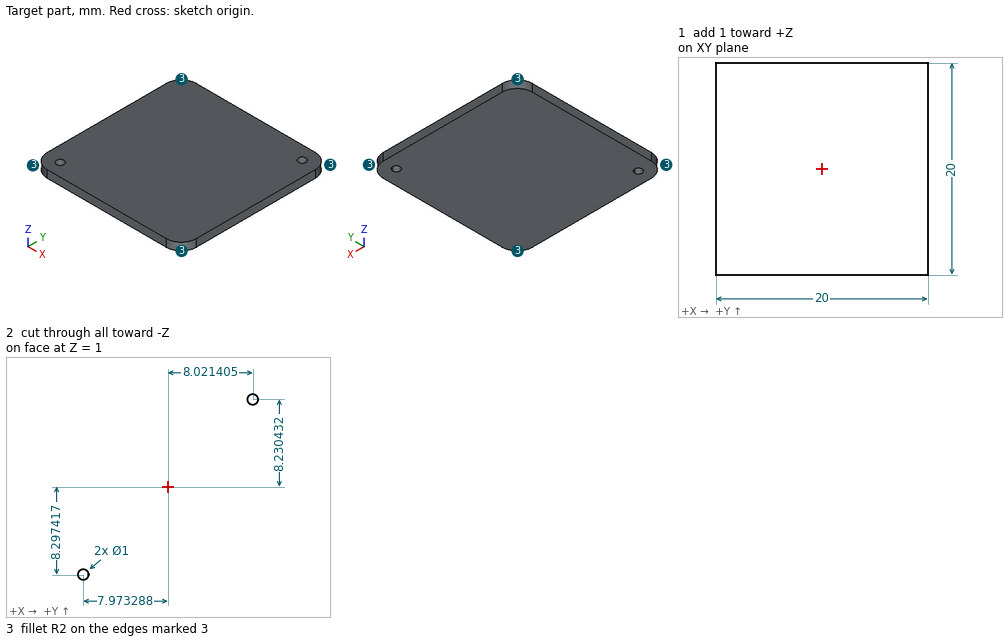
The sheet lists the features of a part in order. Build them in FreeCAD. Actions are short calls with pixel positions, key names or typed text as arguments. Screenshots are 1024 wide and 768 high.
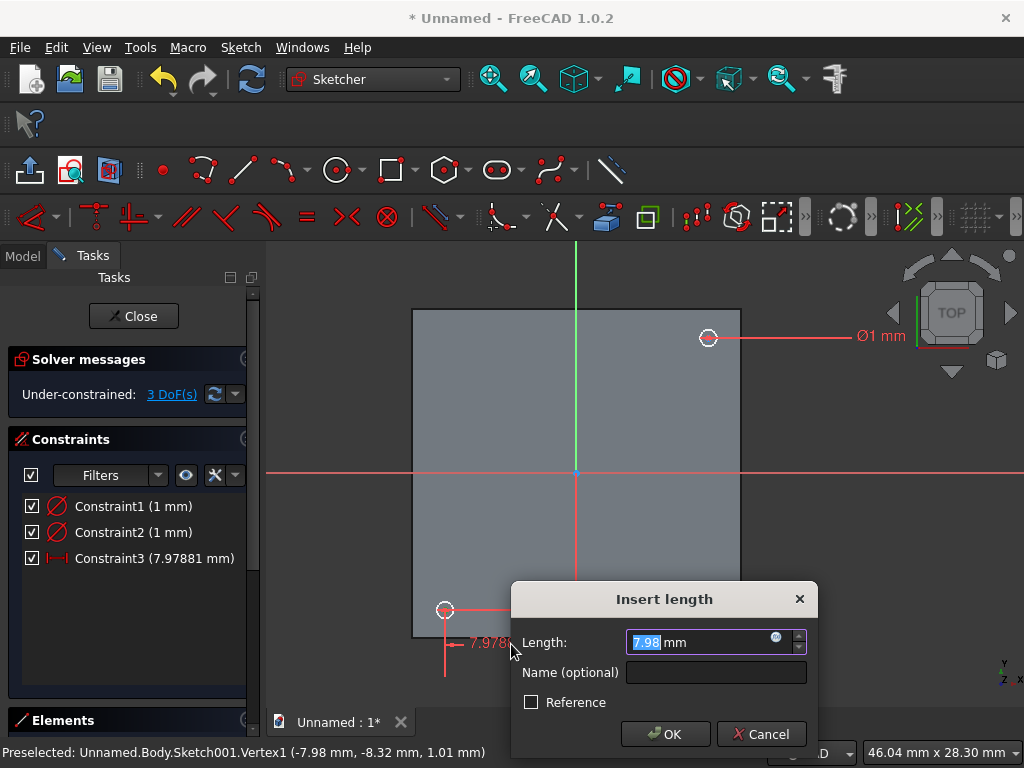
text(7.973288)
key(Return)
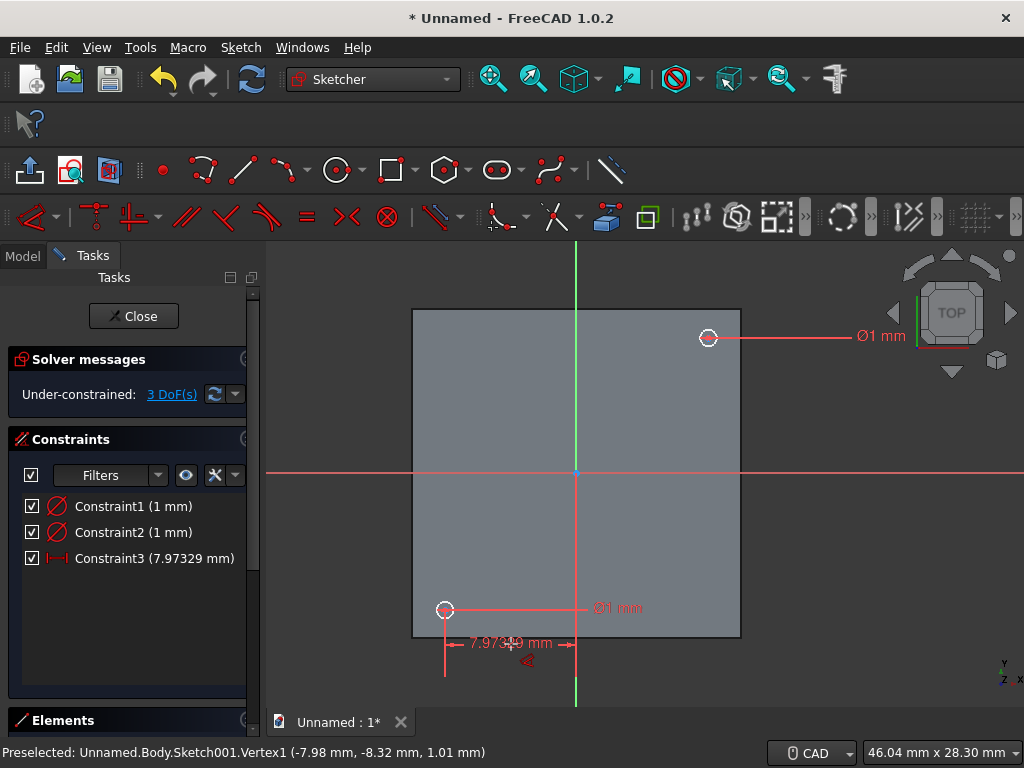
click(445, 610)
click(411, 542)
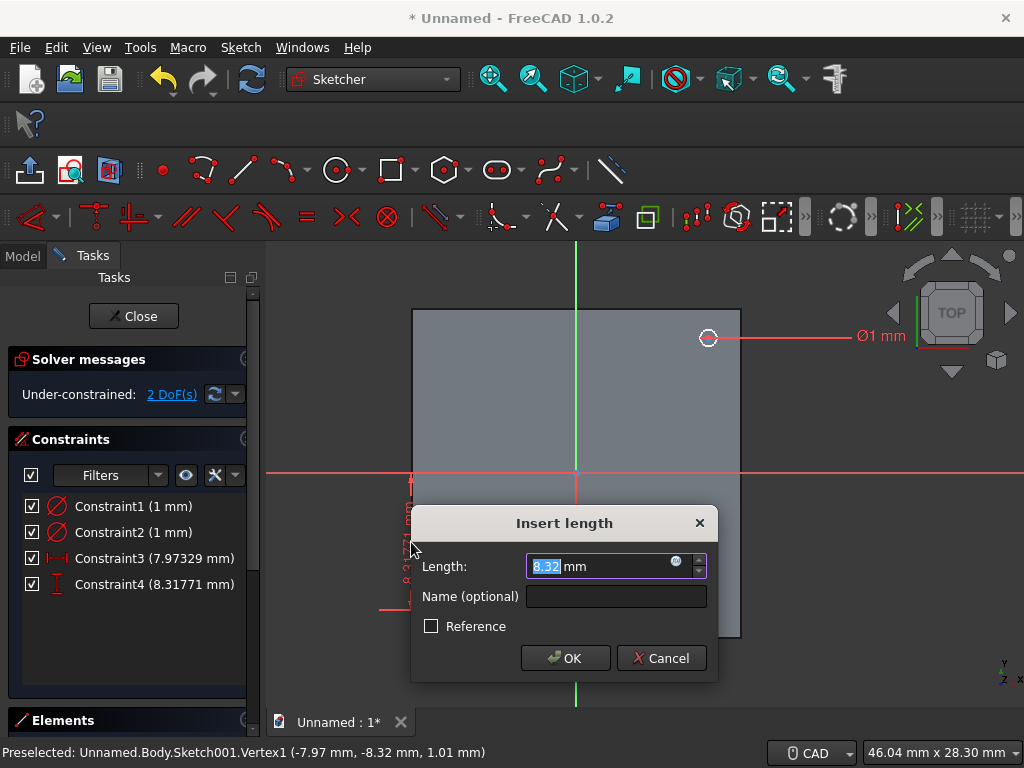
text(8.297417)
key(Return)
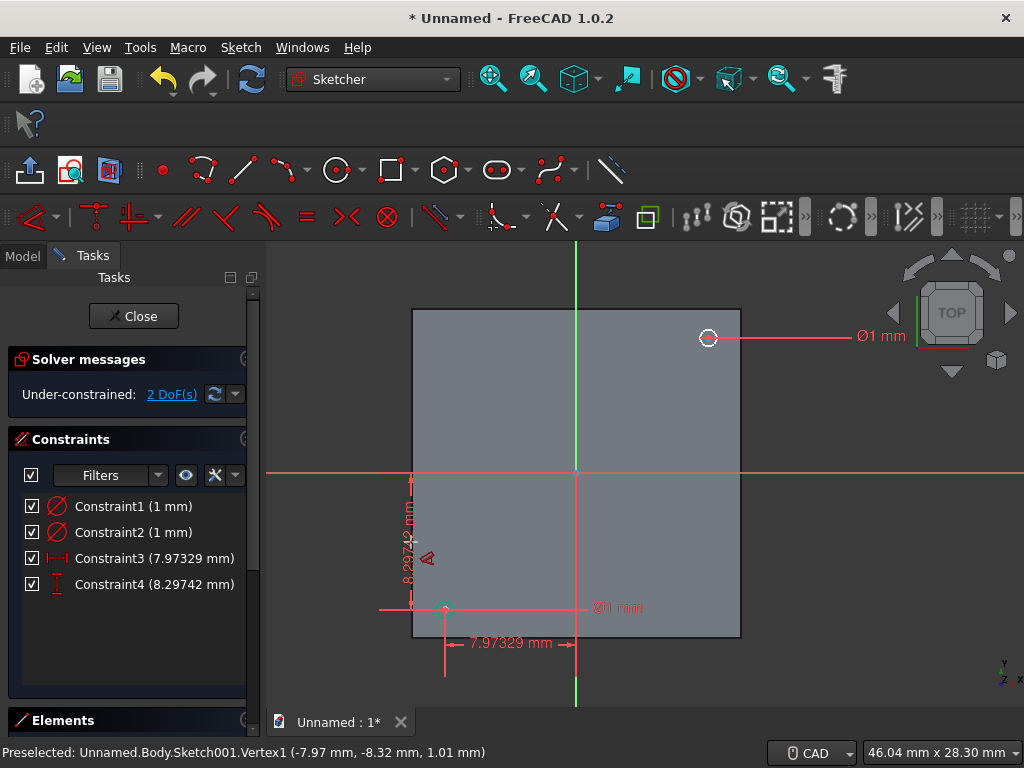
click(709, 338)
click(642, 304)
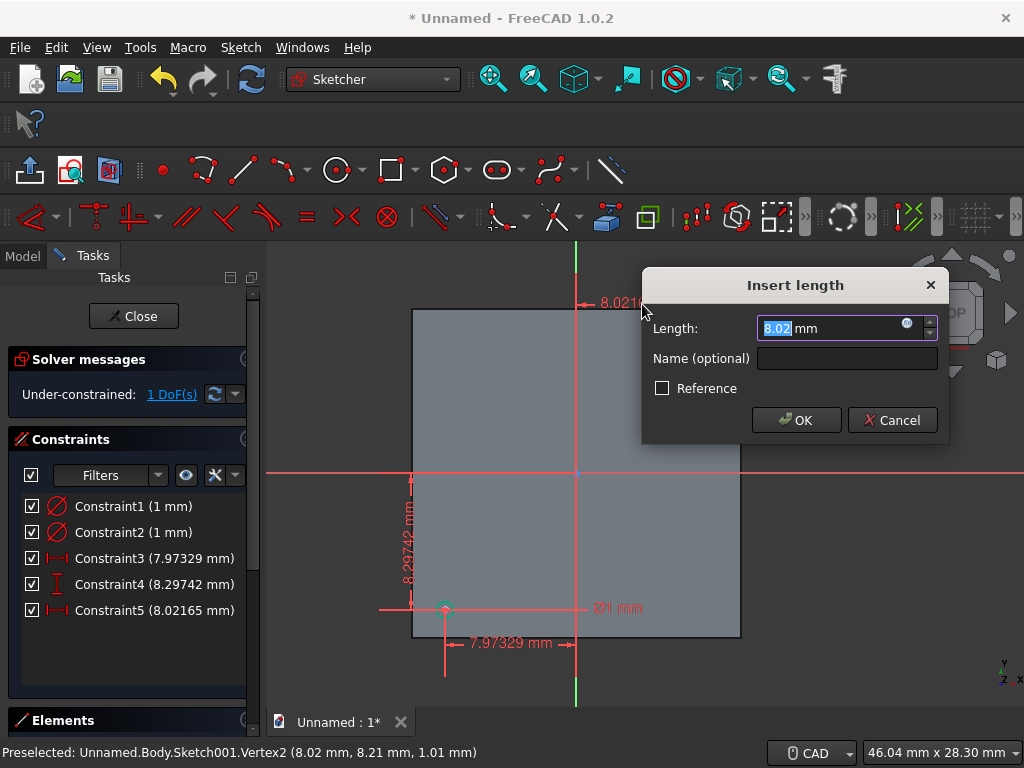
text(8.021405)
key(Return)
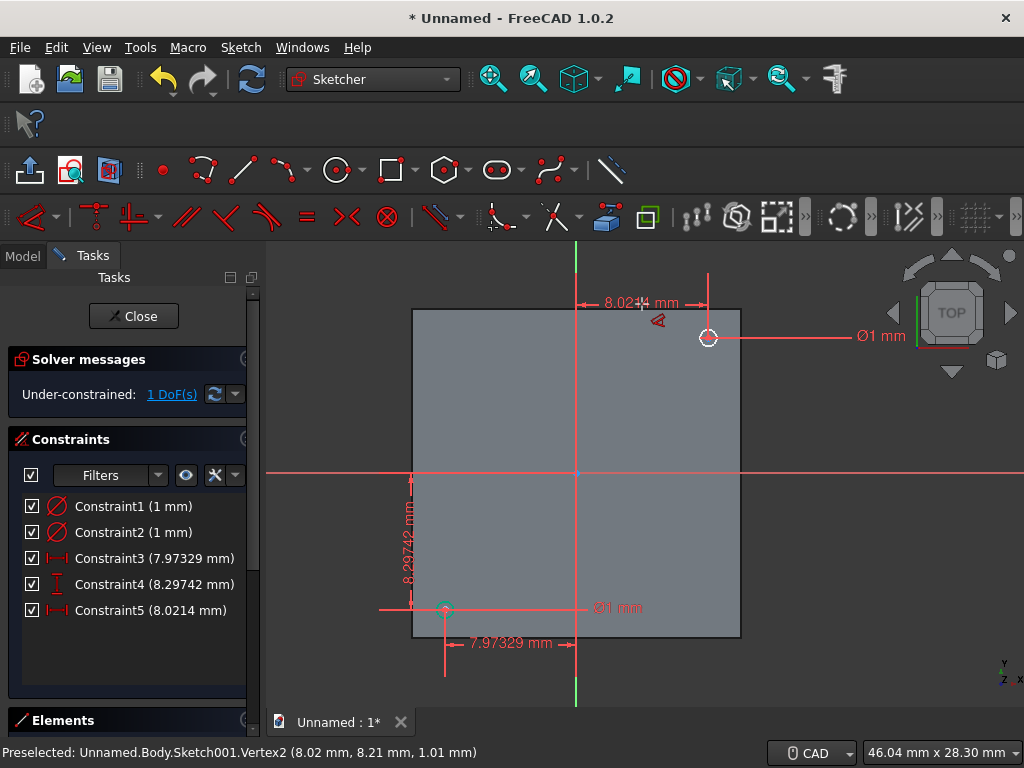
click(709, 338)
click(743, 406)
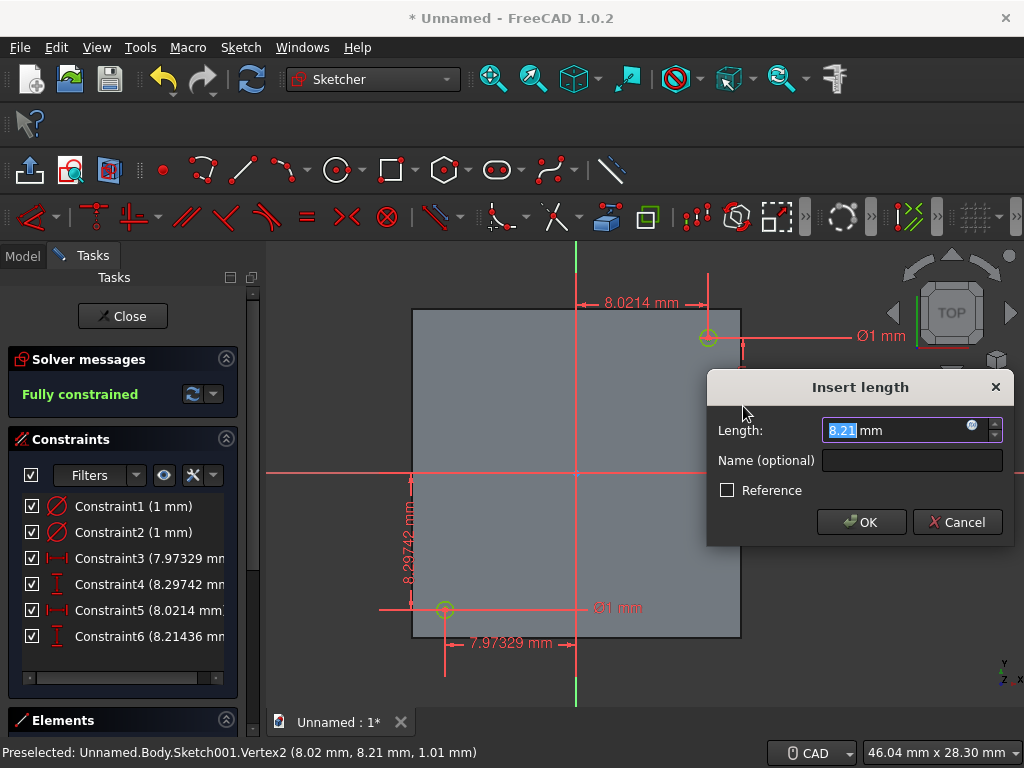
text(8.230432)
key(Return)
key(Escape)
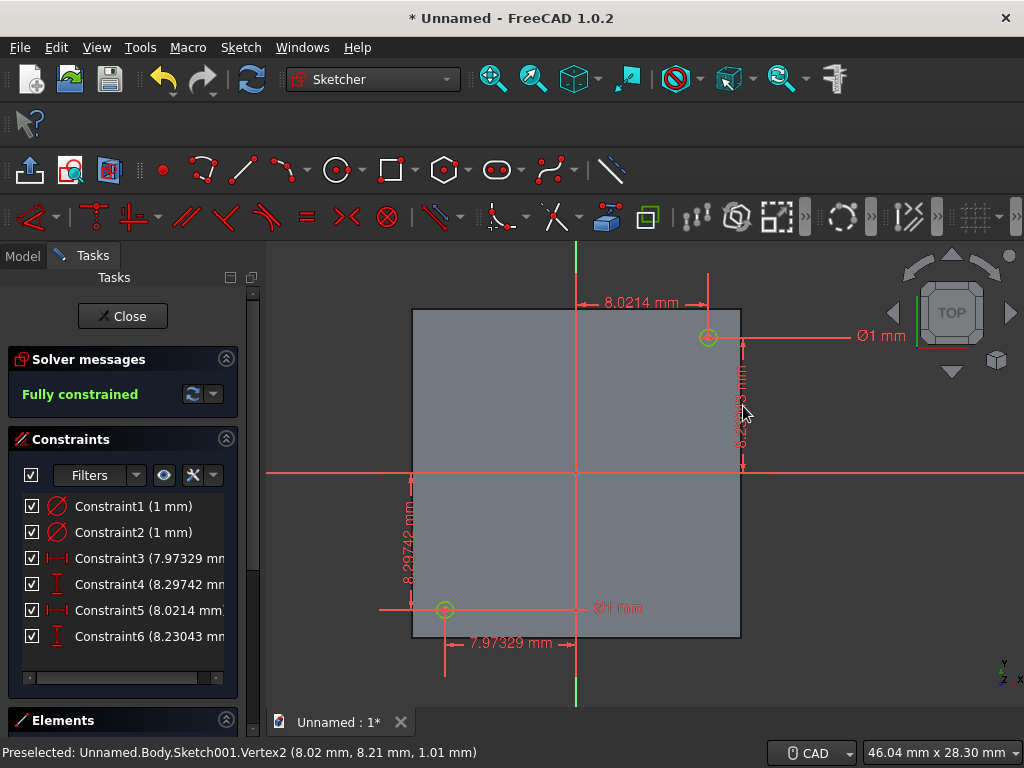
click(123, 316)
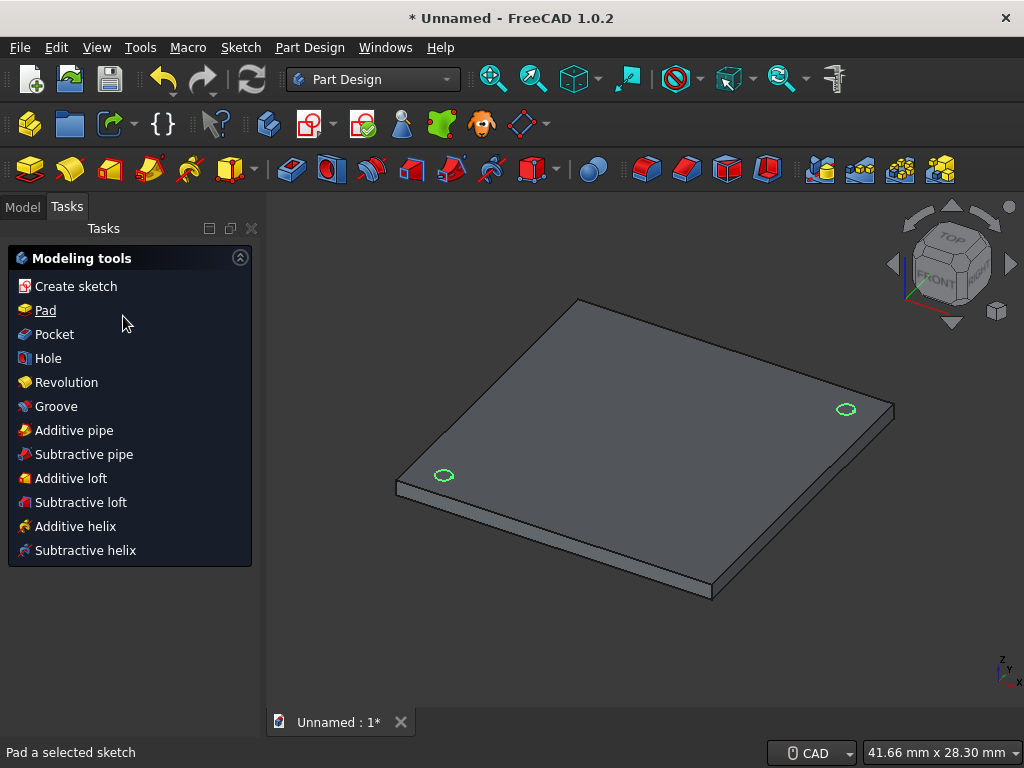
click(292, 170)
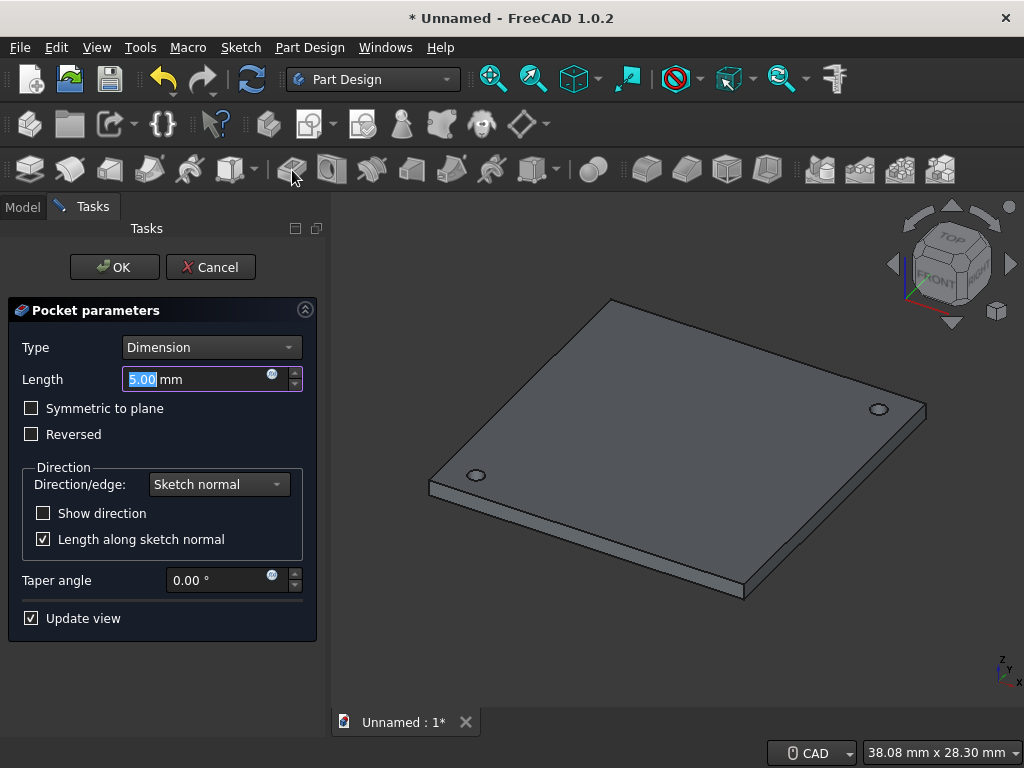
click(212, 348)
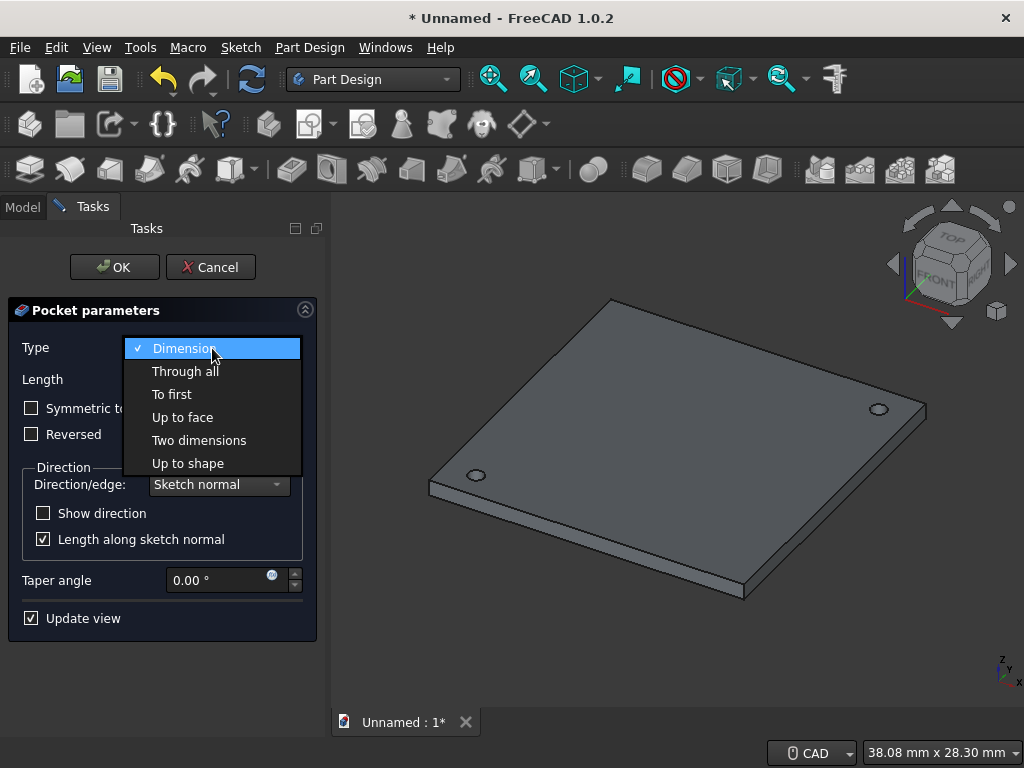
click(212, 372)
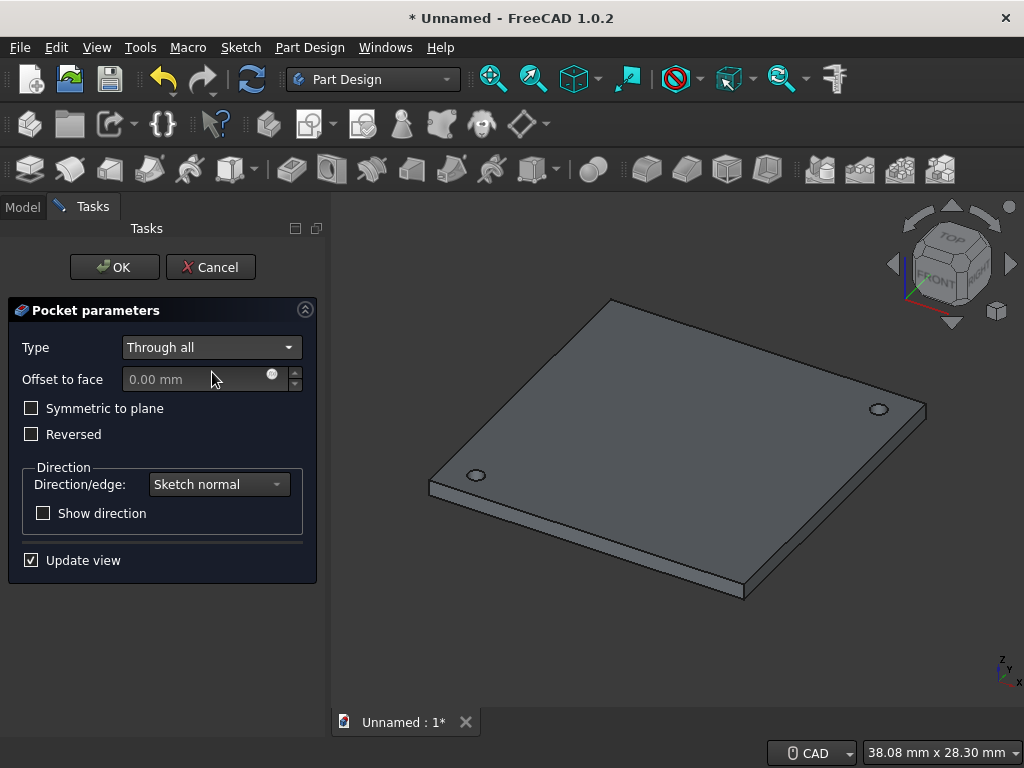
click(115, 267)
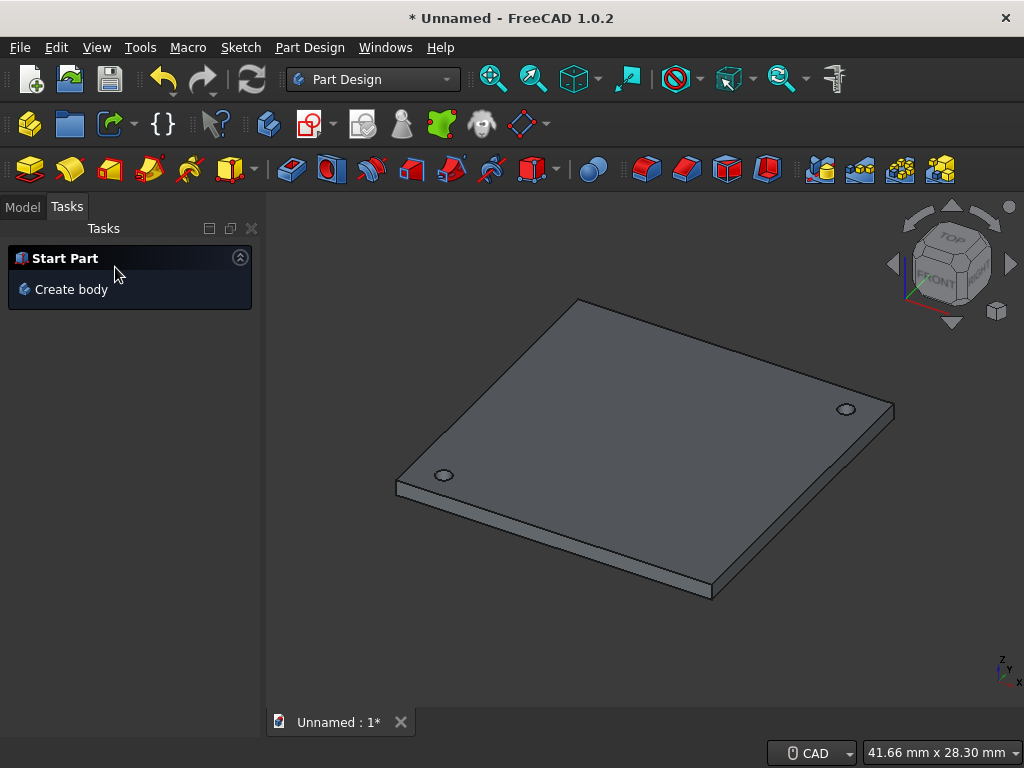
click(712, 591)